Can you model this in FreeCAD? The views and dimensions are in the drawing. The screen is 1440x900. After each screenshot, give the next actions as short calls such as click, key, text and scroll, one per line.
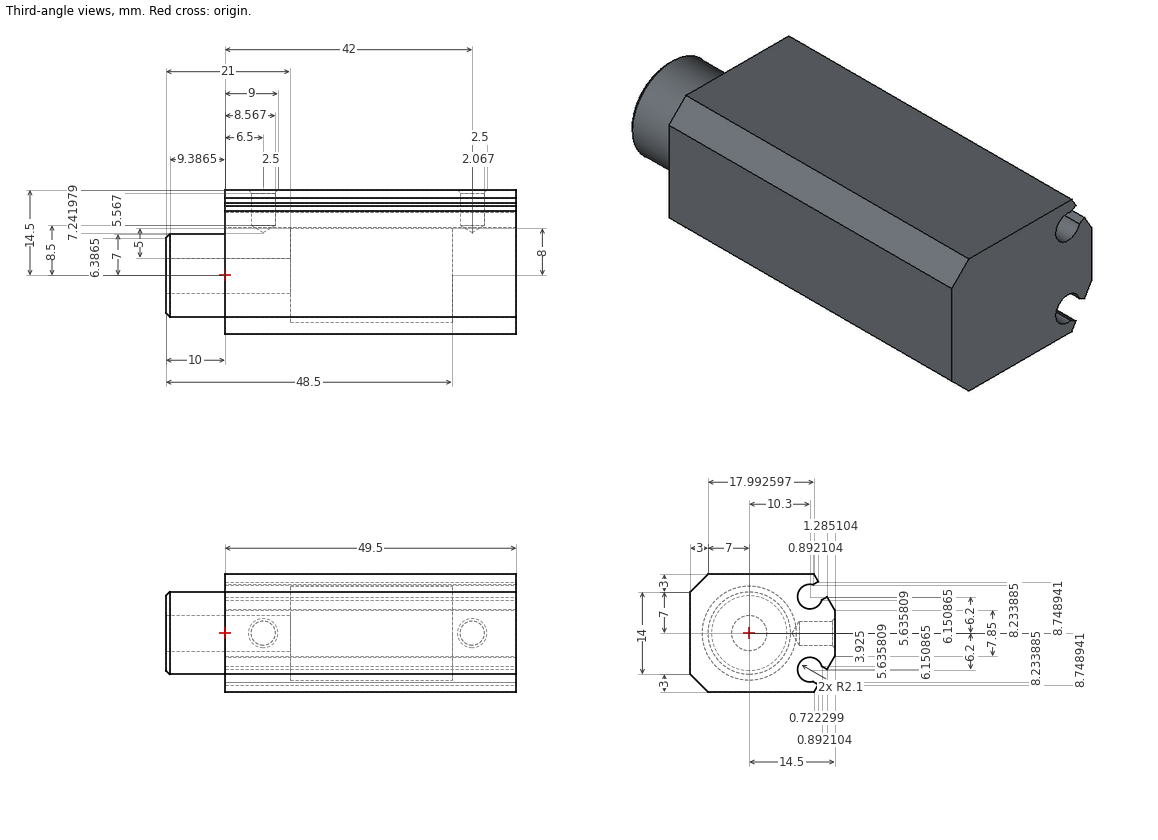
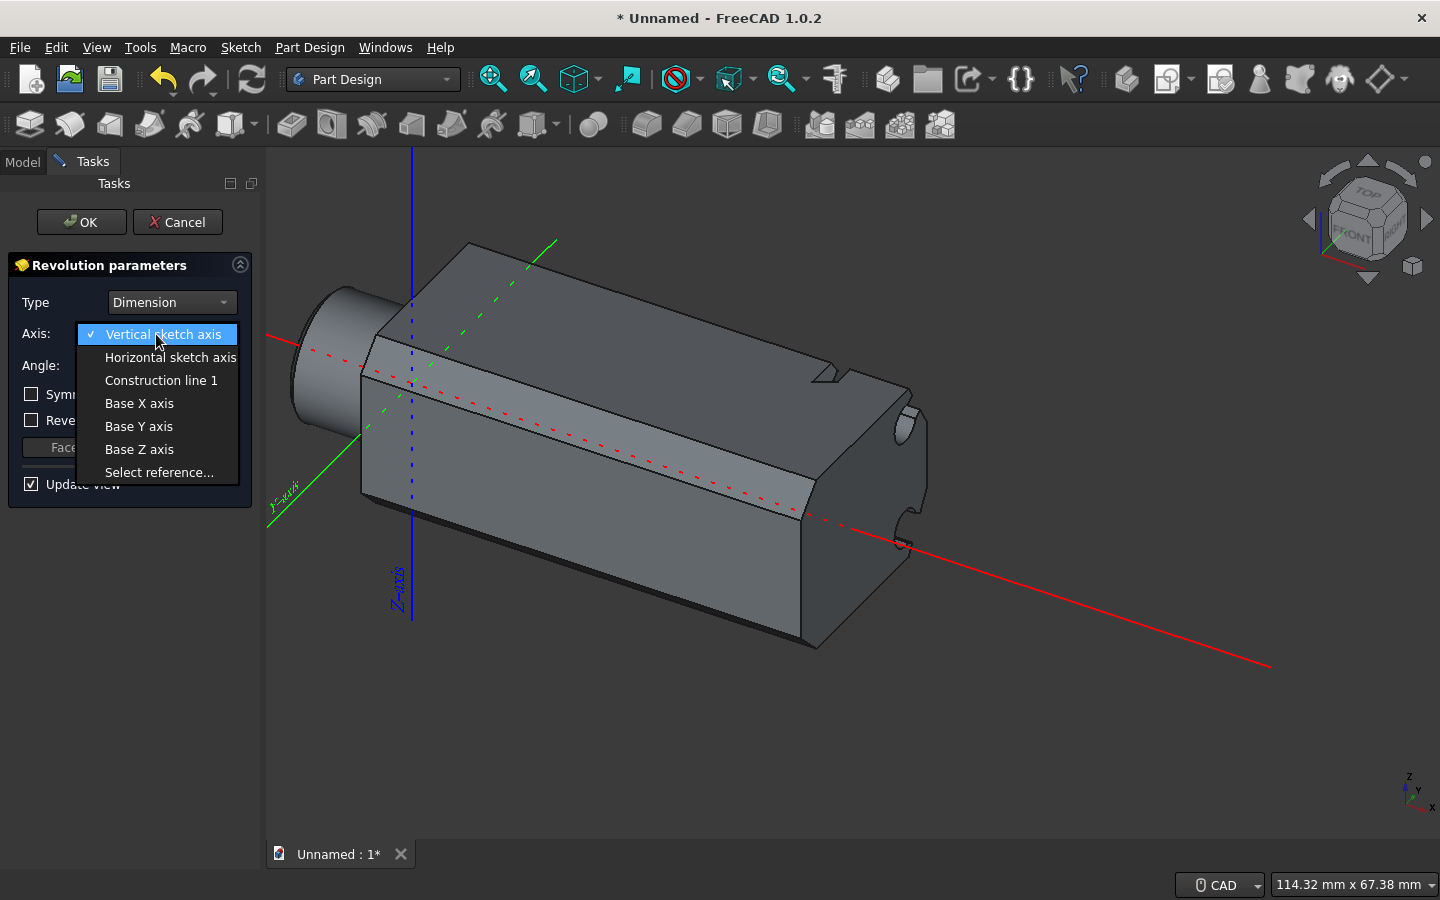
click(156, 380)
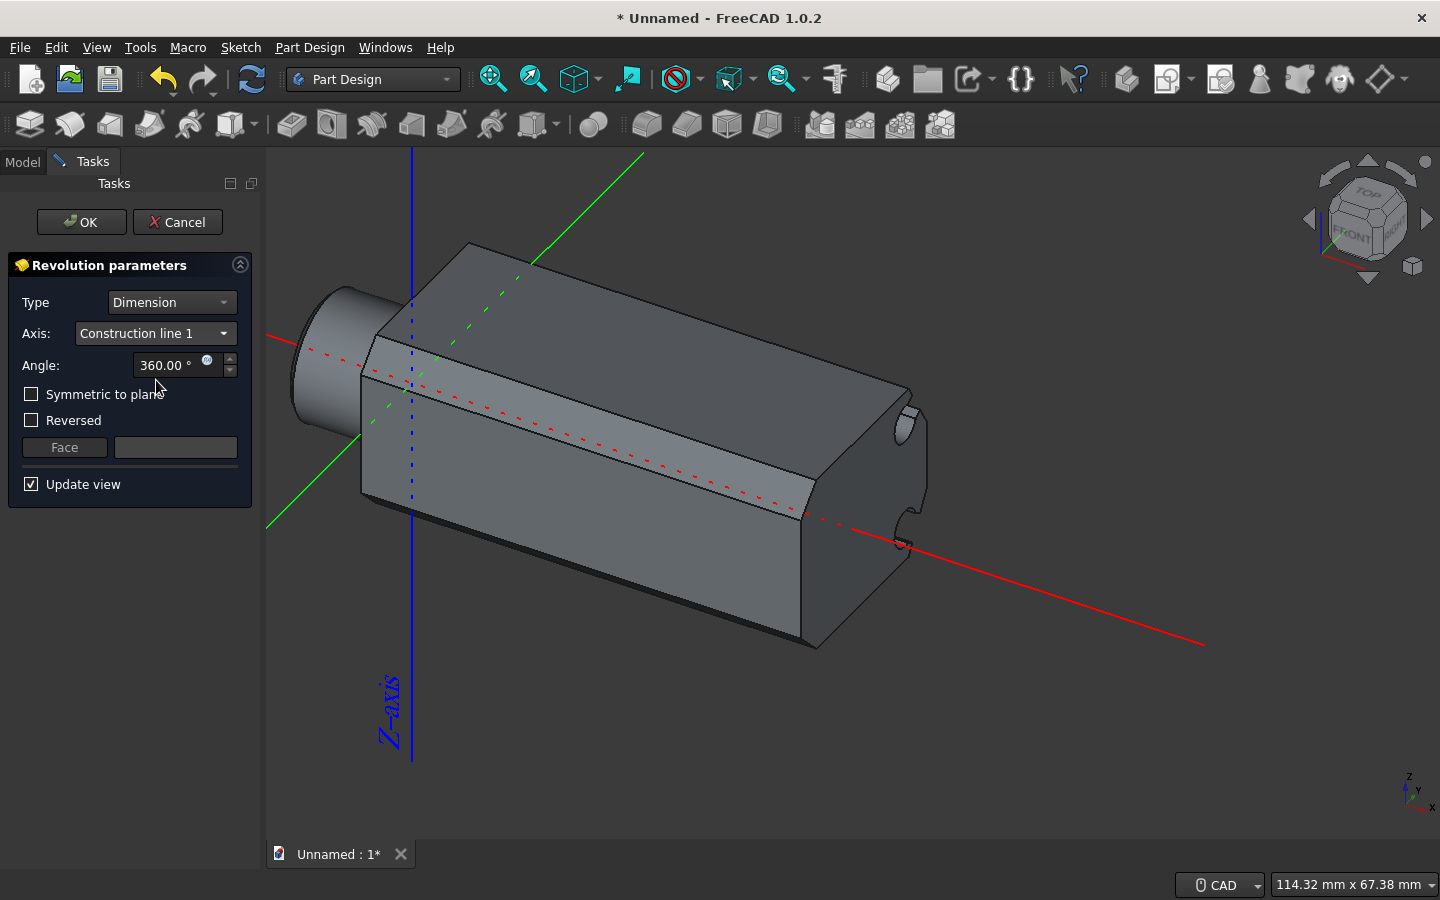
click(82, 222)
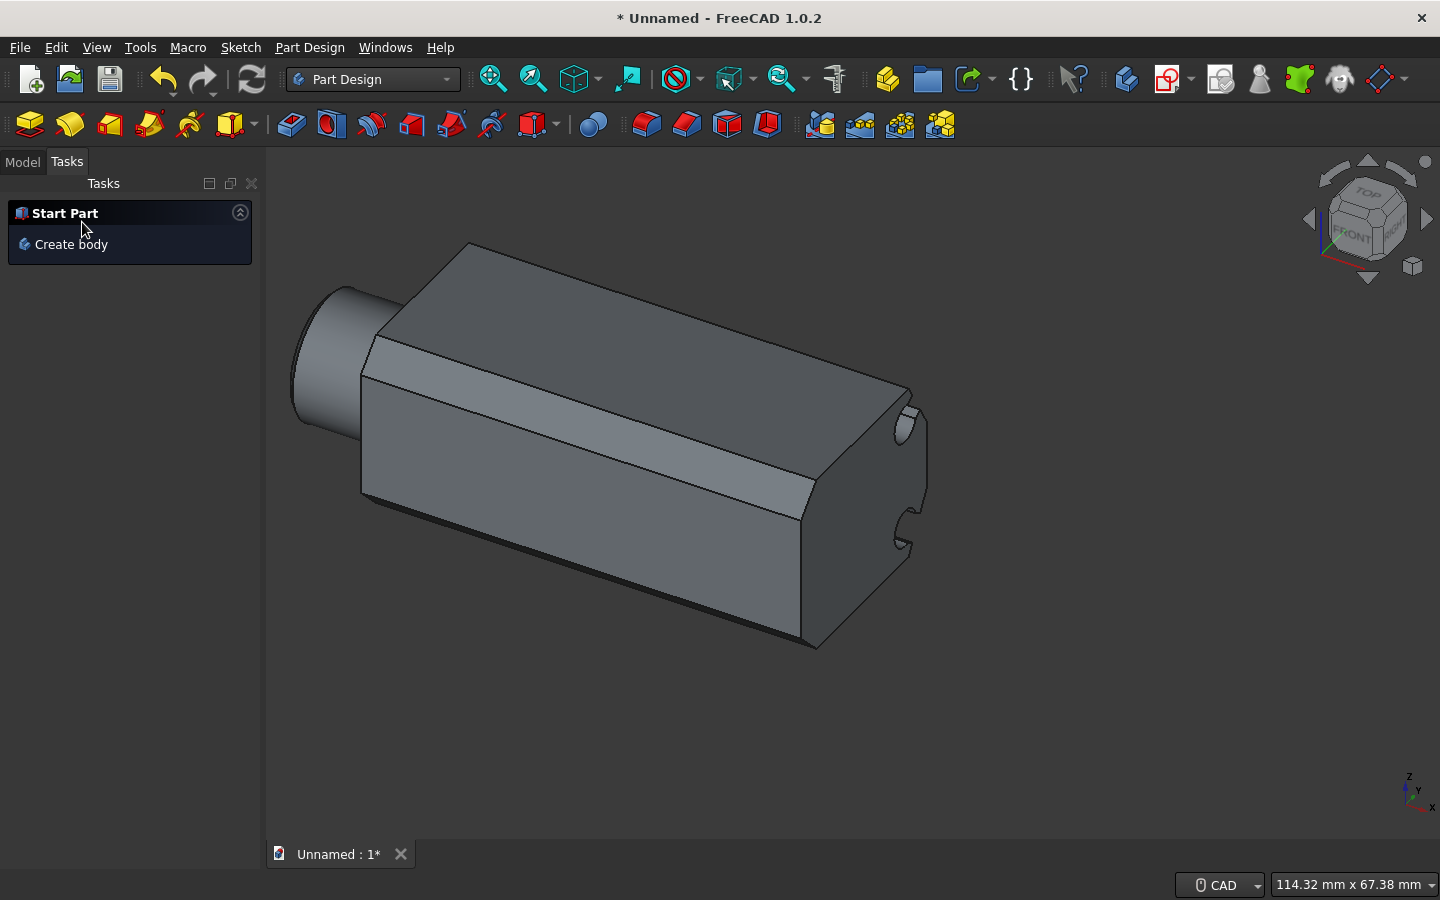
key(0)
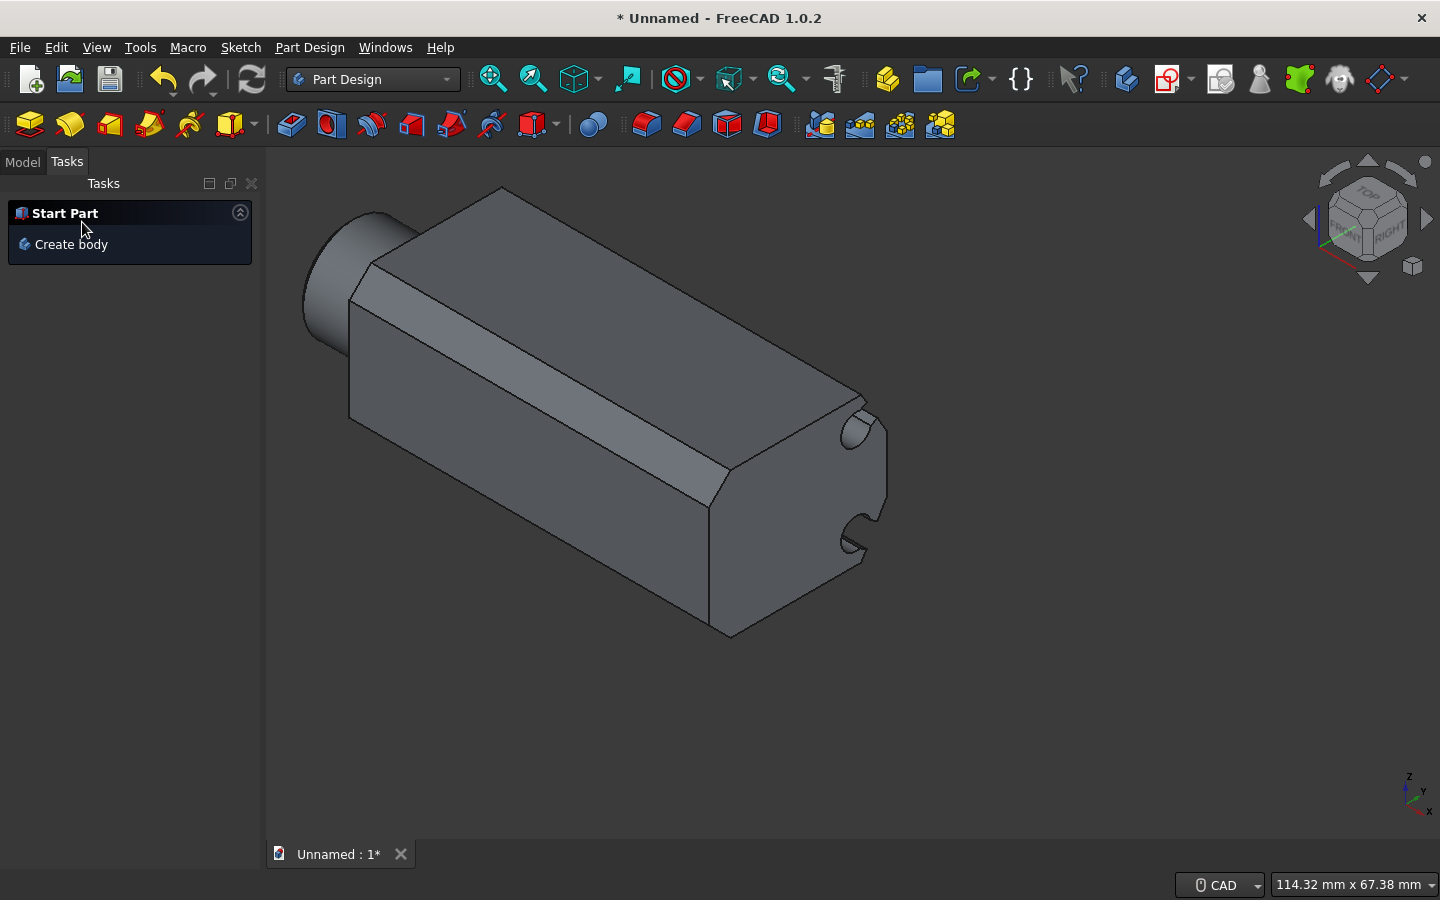
click(494, 80)